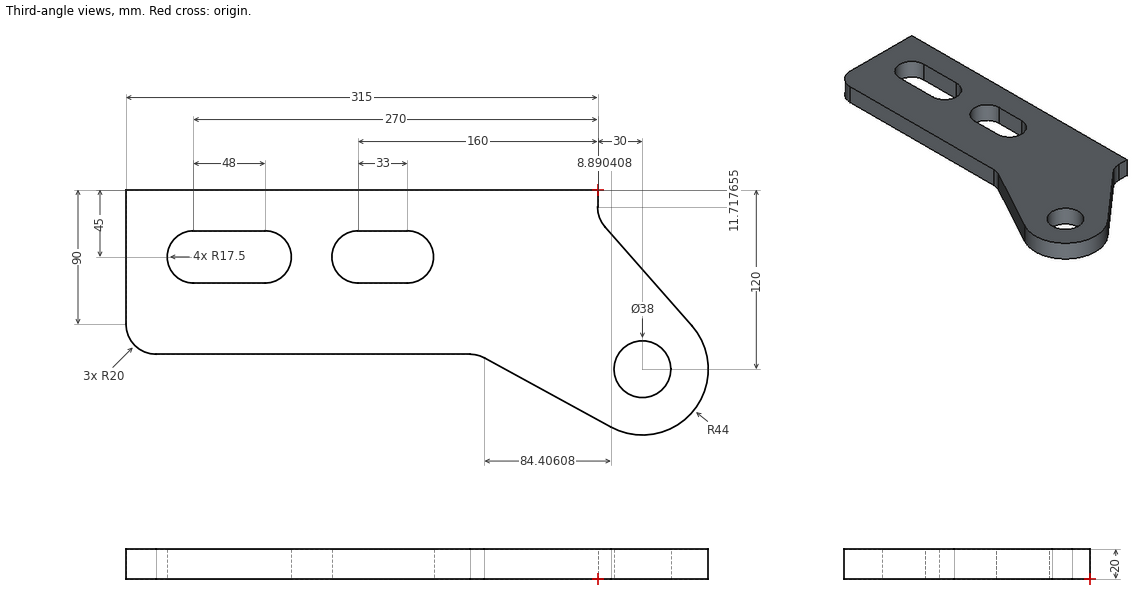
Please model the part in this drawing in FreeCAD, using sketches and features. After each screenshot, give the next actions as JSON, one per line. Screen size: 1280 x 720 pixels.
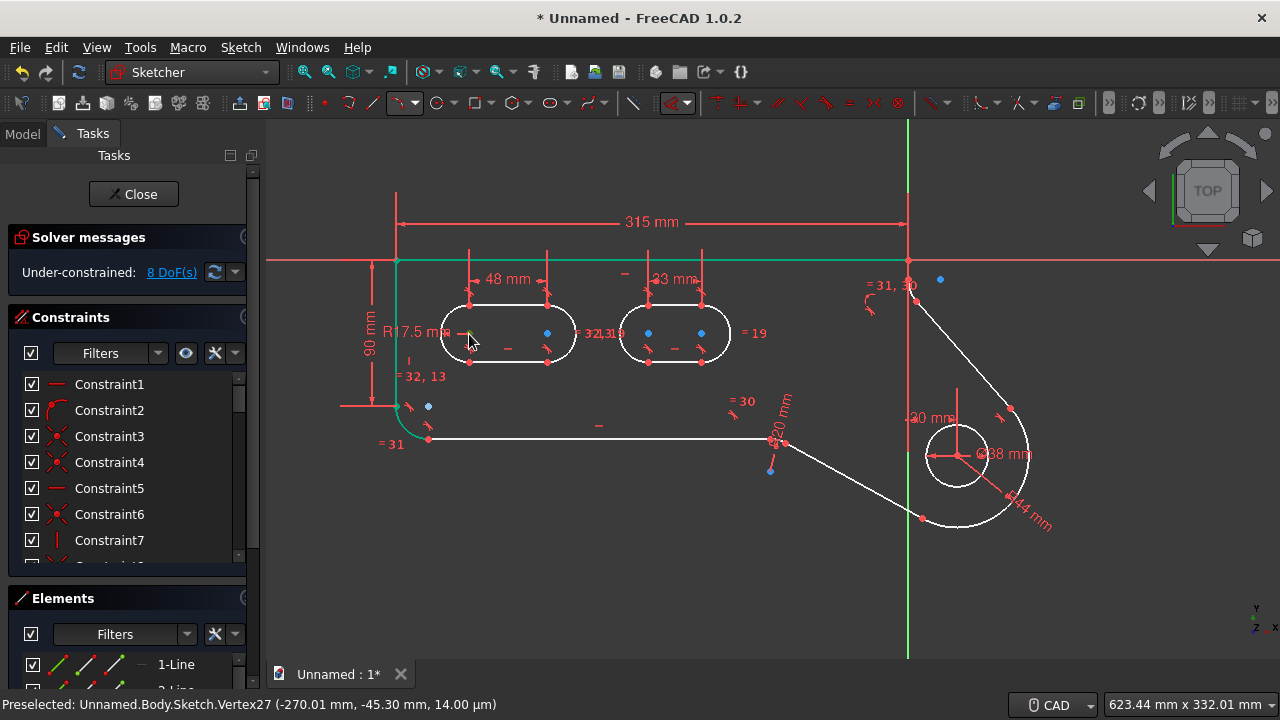
{"action": "key", "text": "i"}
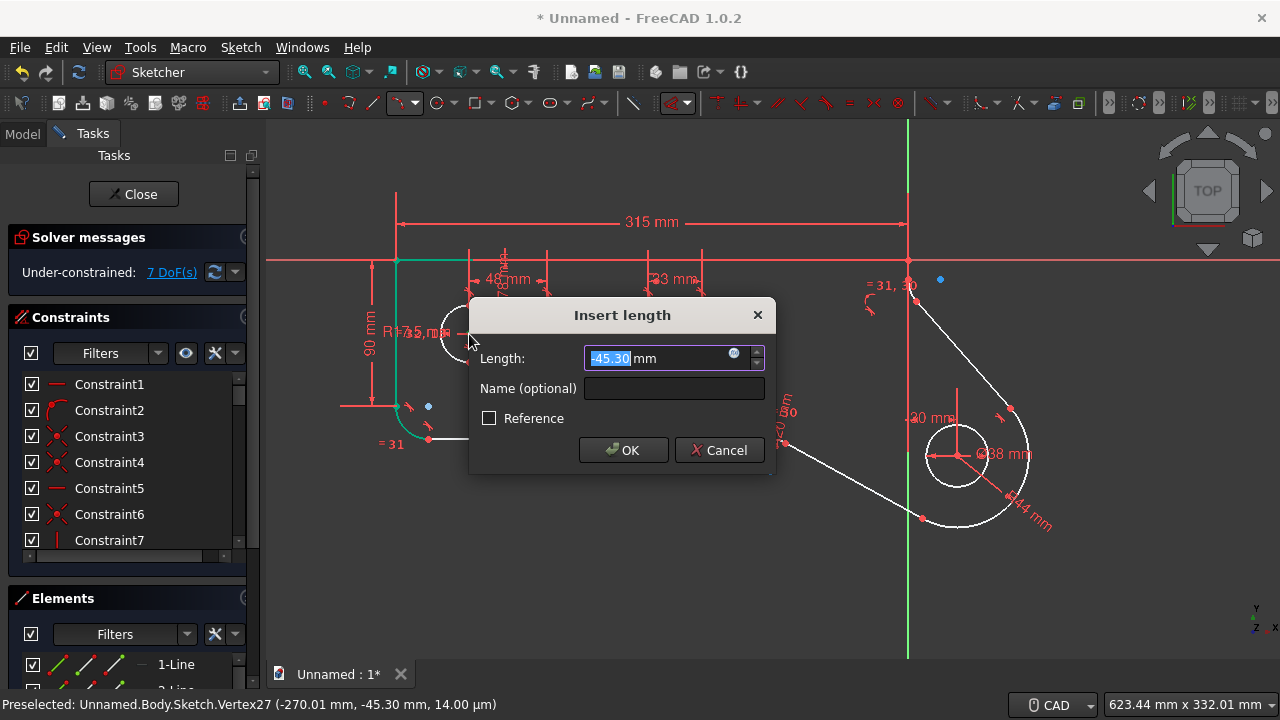
{"action": "type", "text": "-45"}
{"action": "key", "text": "Return"}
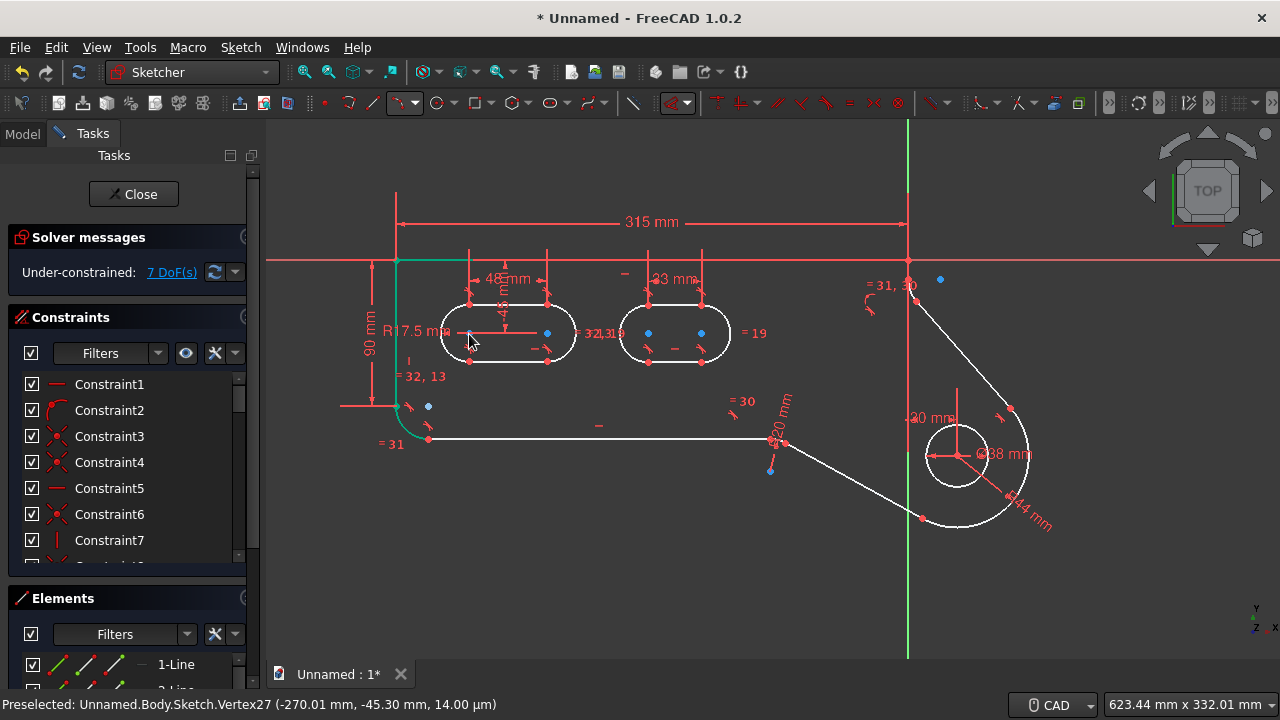
{"action": "left_click", "coordinate": [648, 334]}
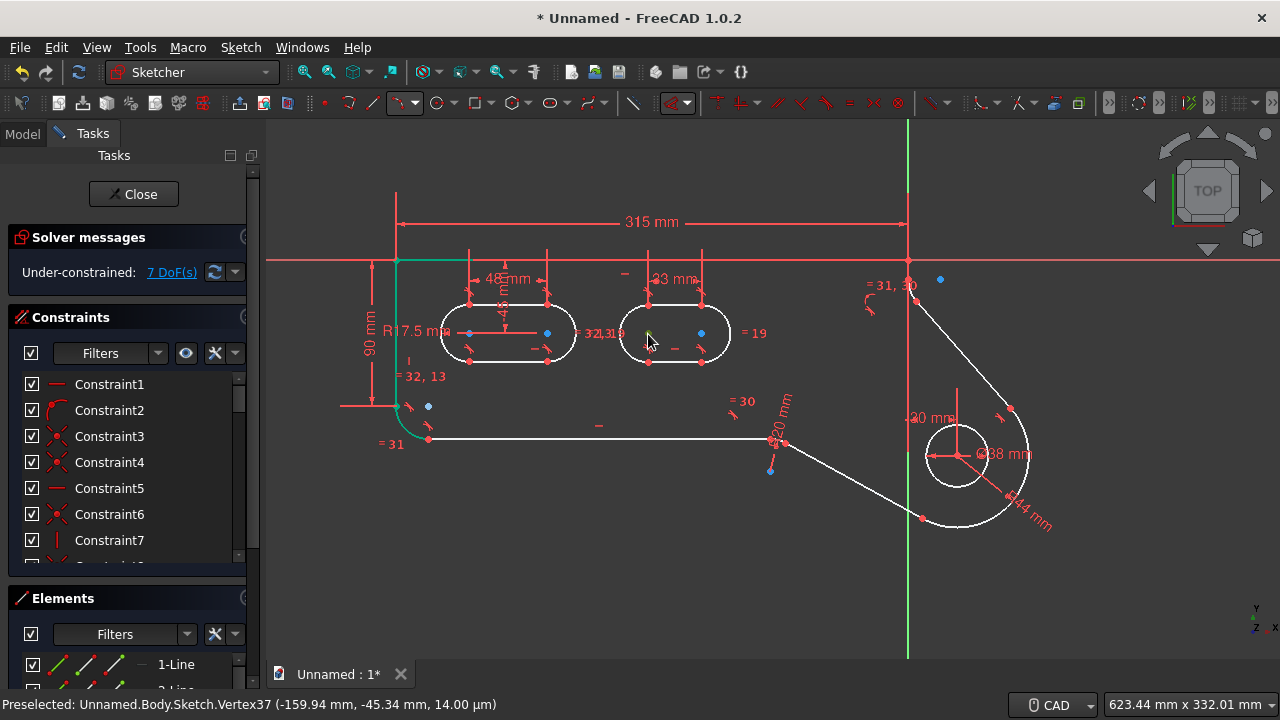
{"action": "left_click", "coordinate": [690, 104]}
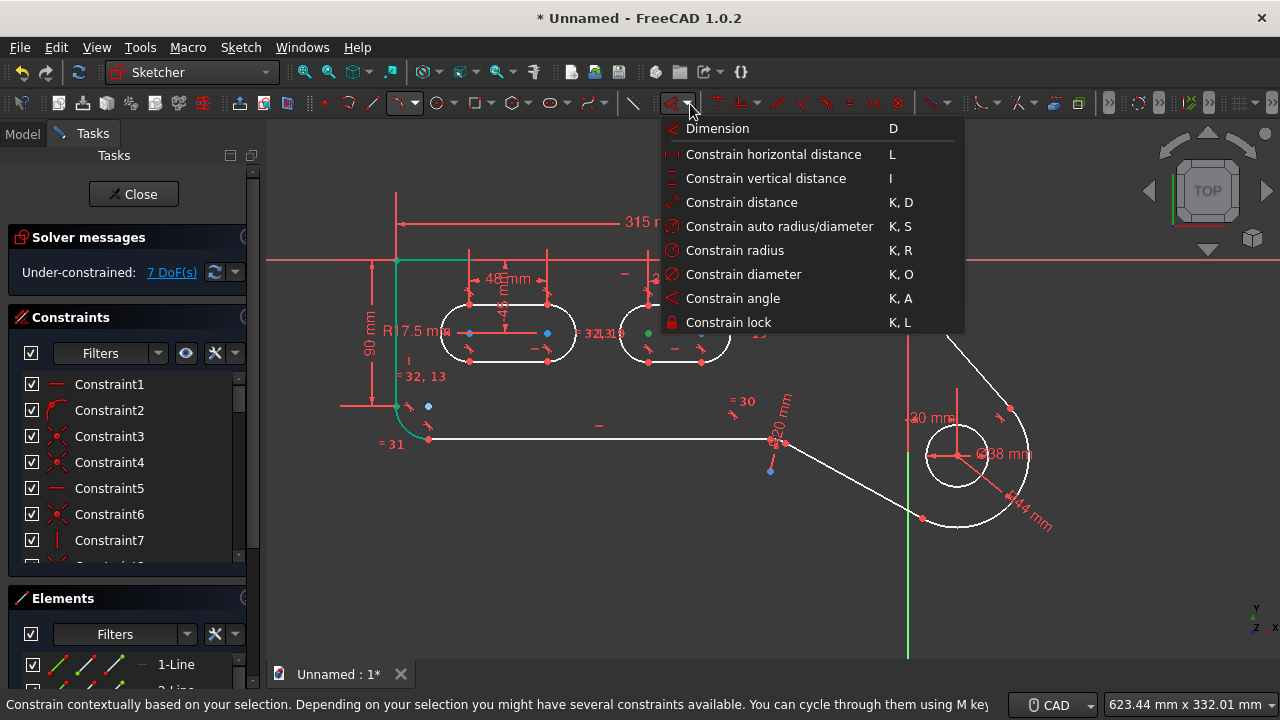
{"action": "left_click", "coordinate": [813, 178]}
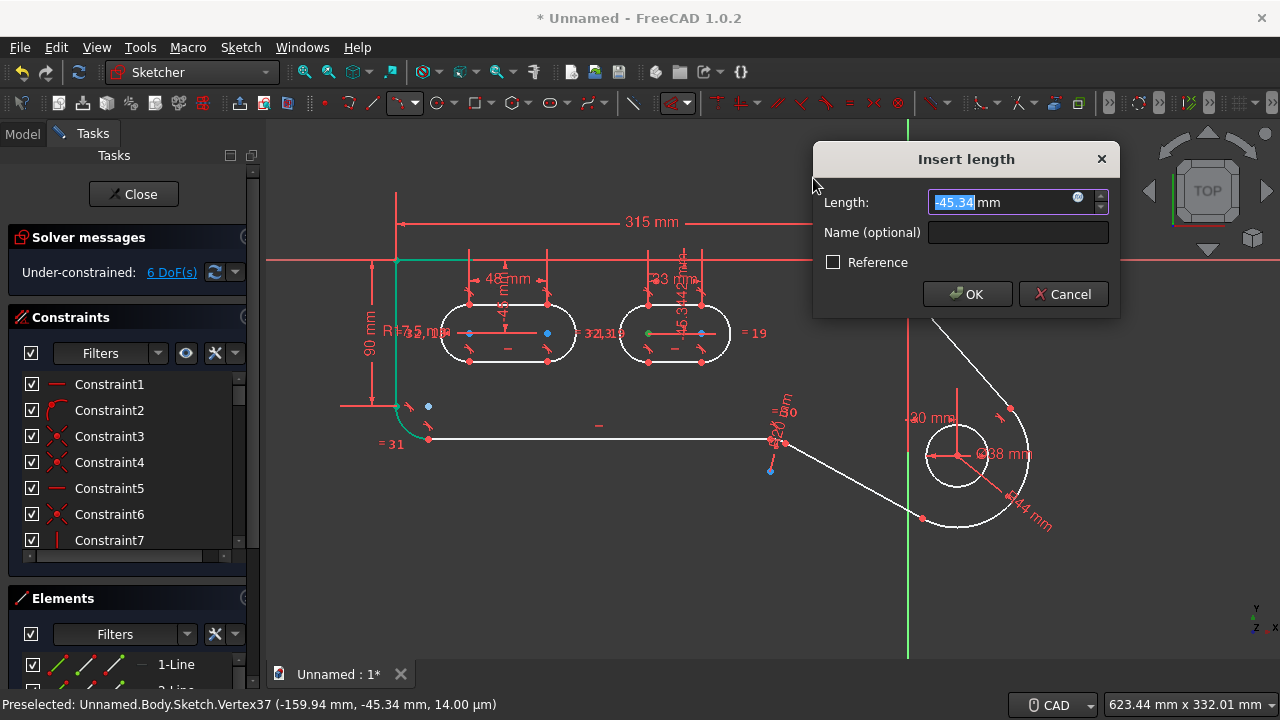
{"action": "type", "text": "-45"}
{"action": "key", "text": "Return"}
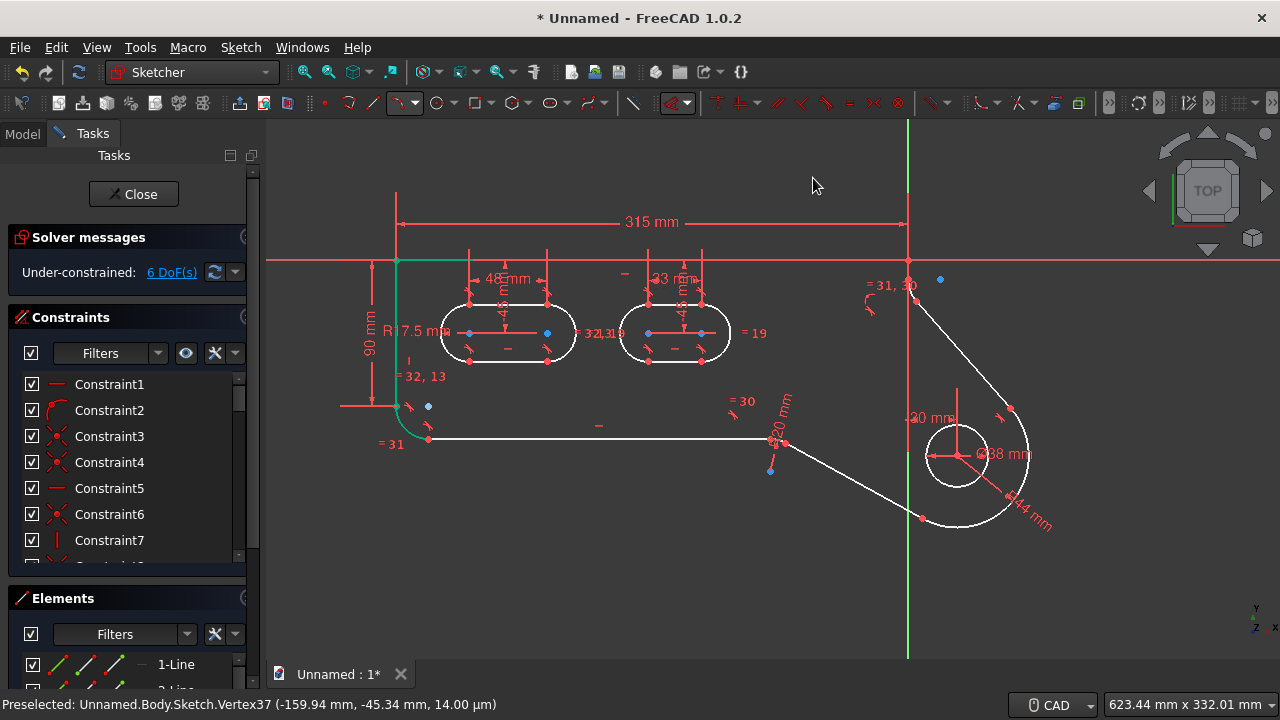
{"action": "left_click", "coordinate": [957, 456]}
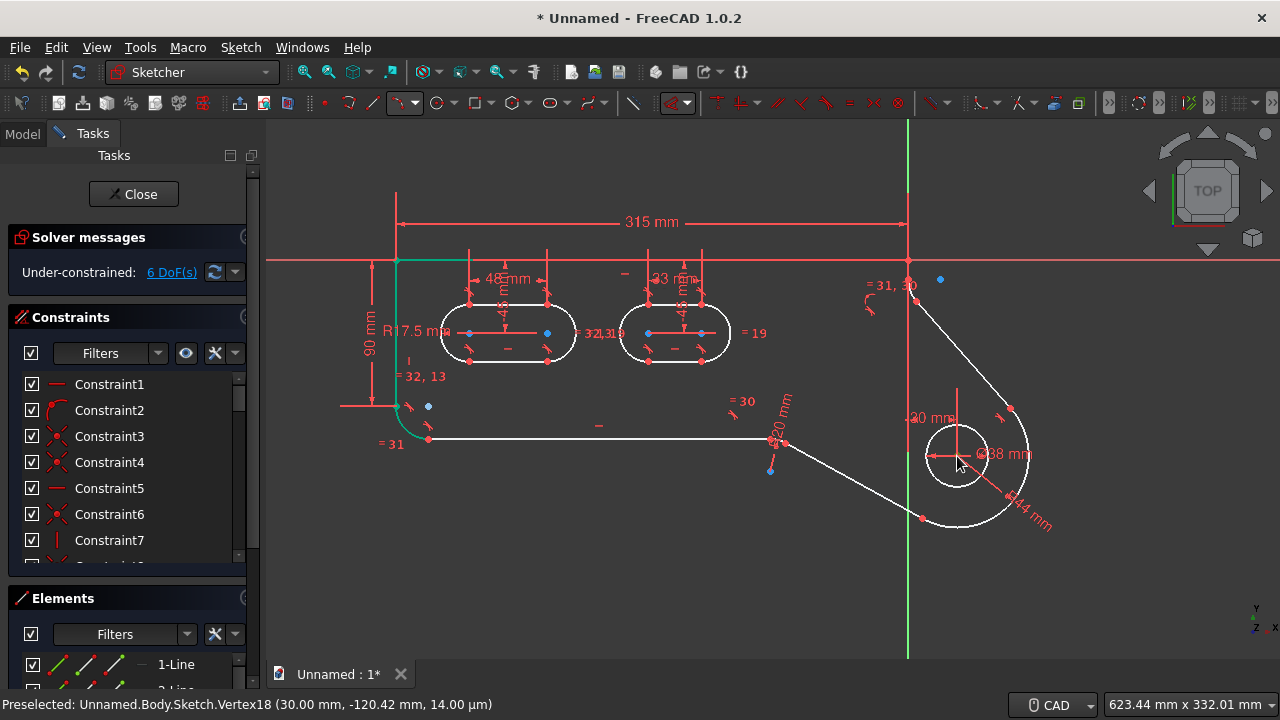
{"action": "left_click", "coordinate": [690, 104]}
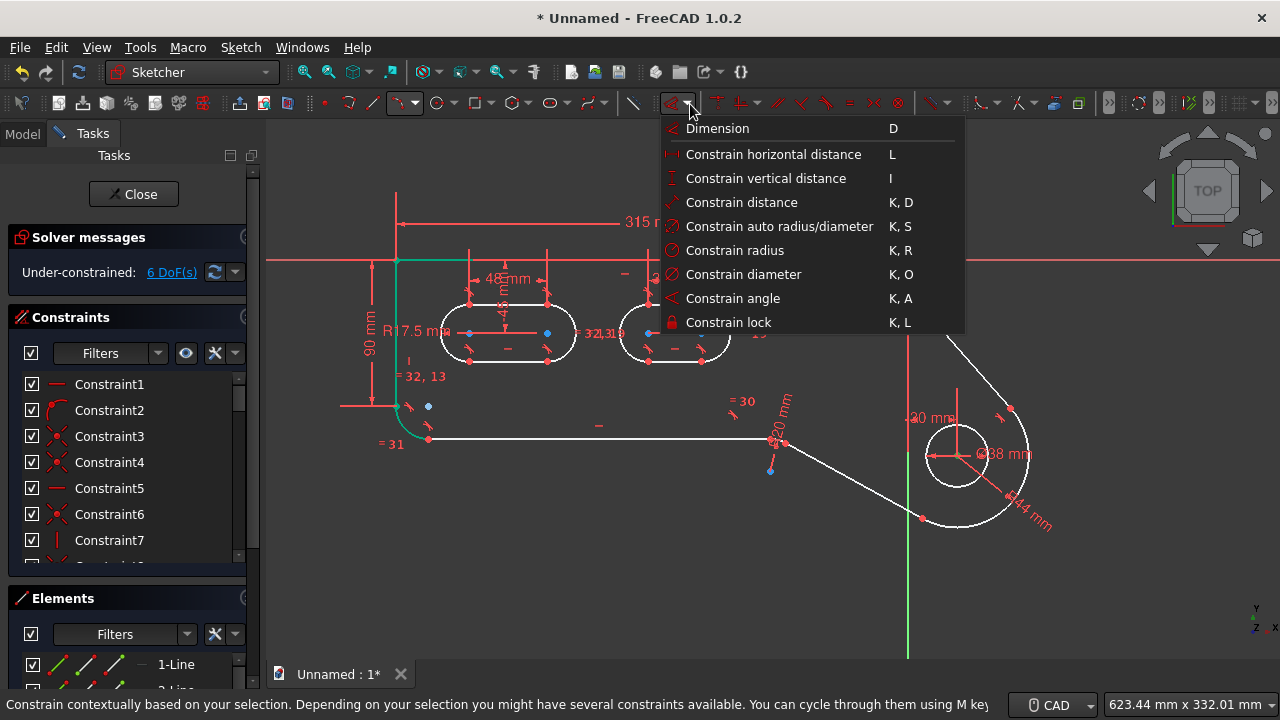
{"action": "left_click", "coordinate": [813, 178]}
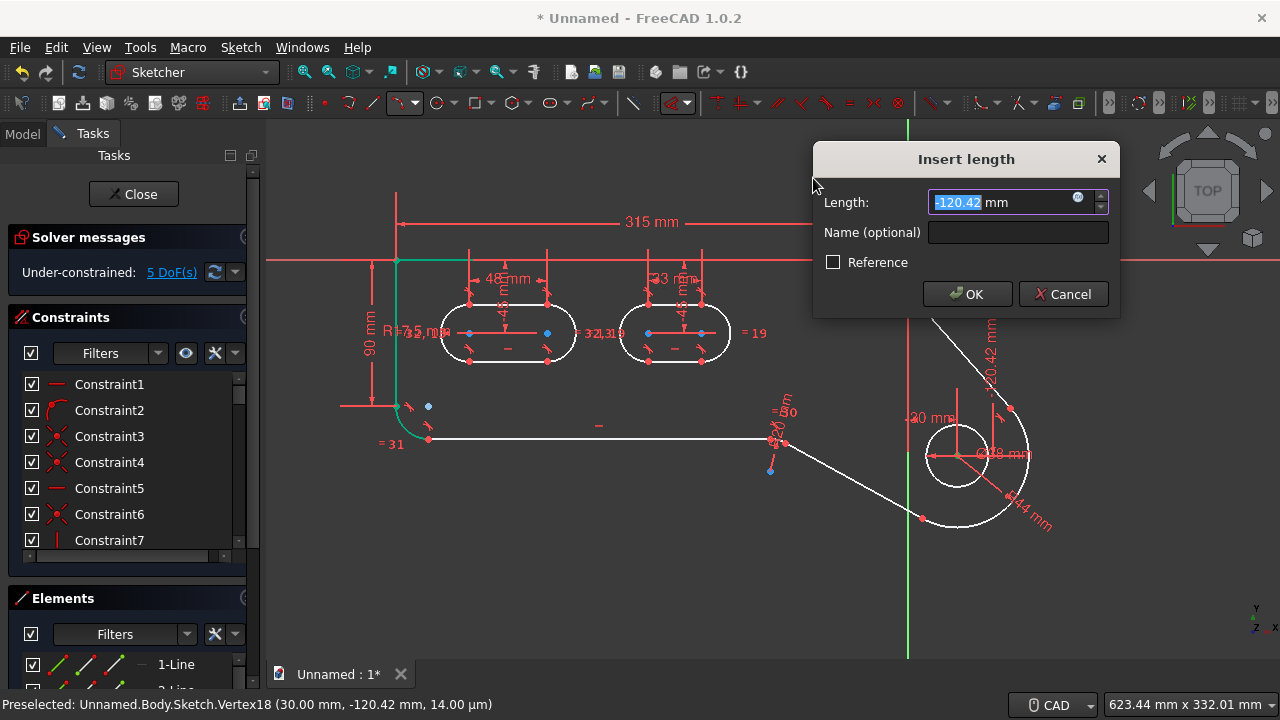
{"action": "type", "text": "-120"}
{"action": "key", "text": "Return"}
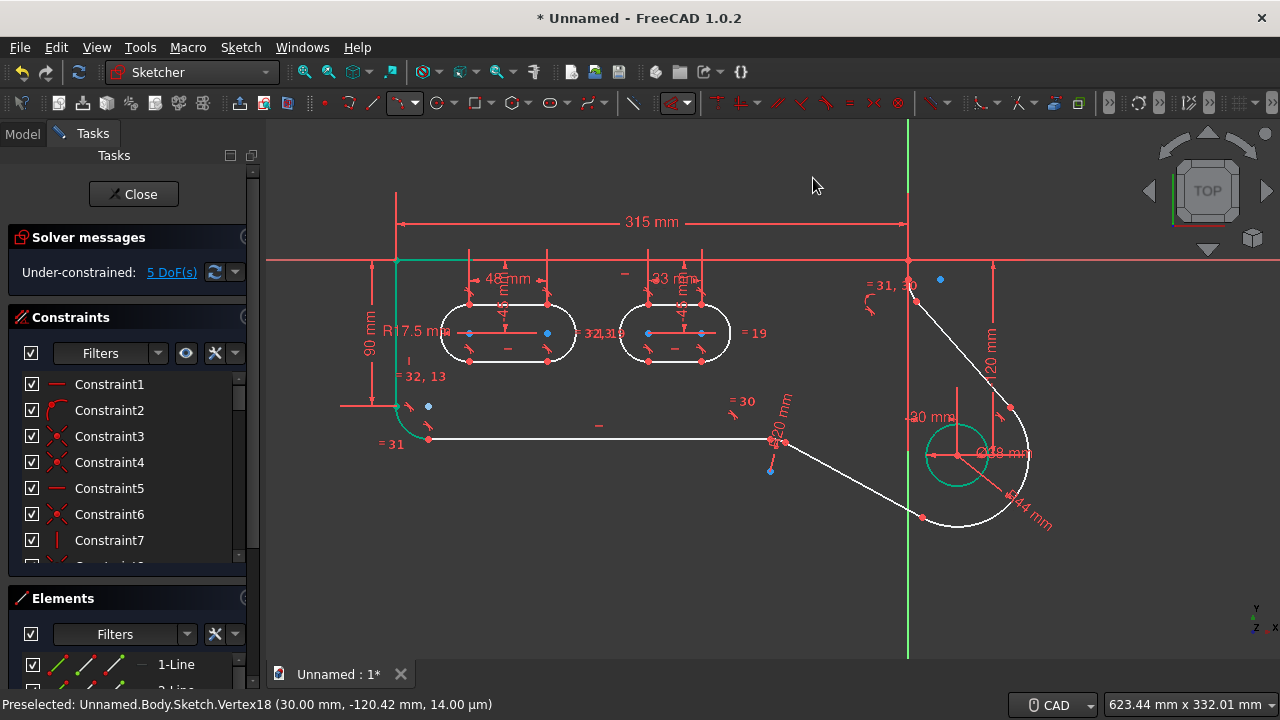
{"action": "left_click", "coordinate": [469, 305]}